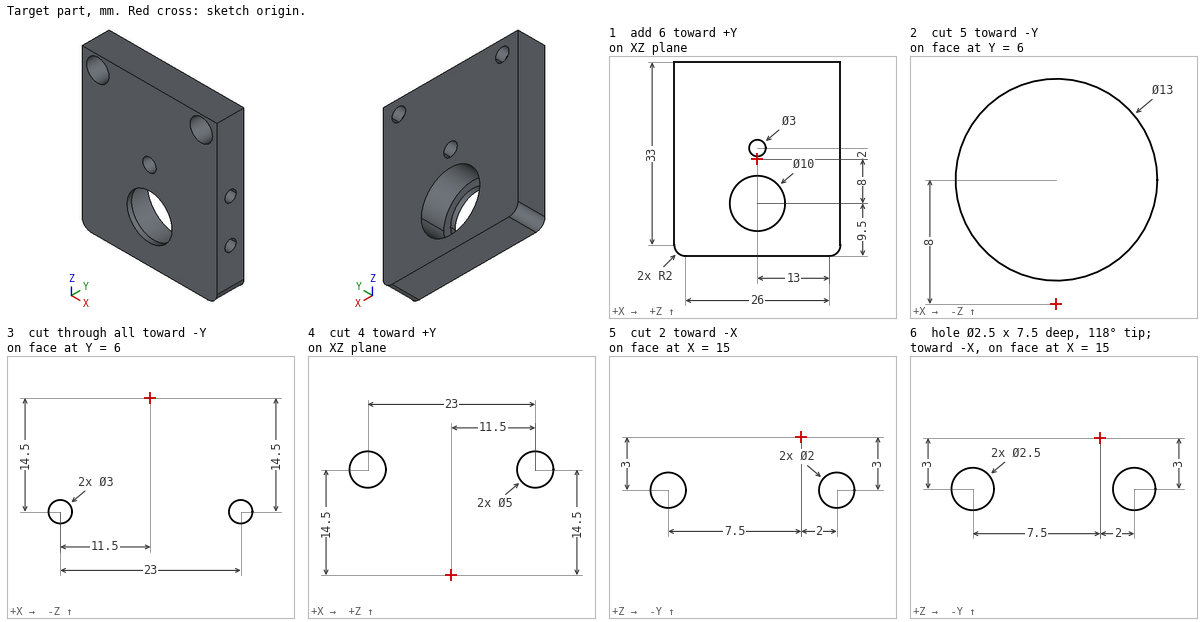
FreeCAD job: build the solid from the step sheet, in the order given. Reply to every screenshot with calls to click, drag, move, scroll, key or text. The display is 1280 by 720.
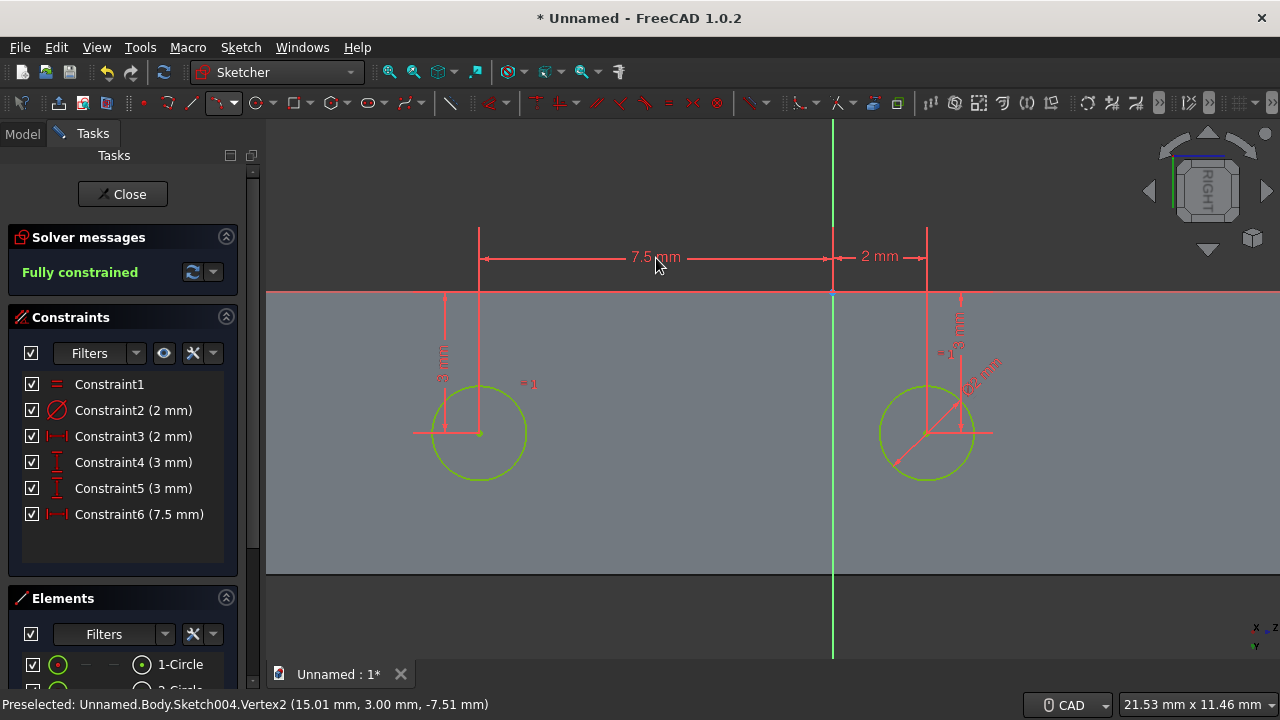
click(123, 194)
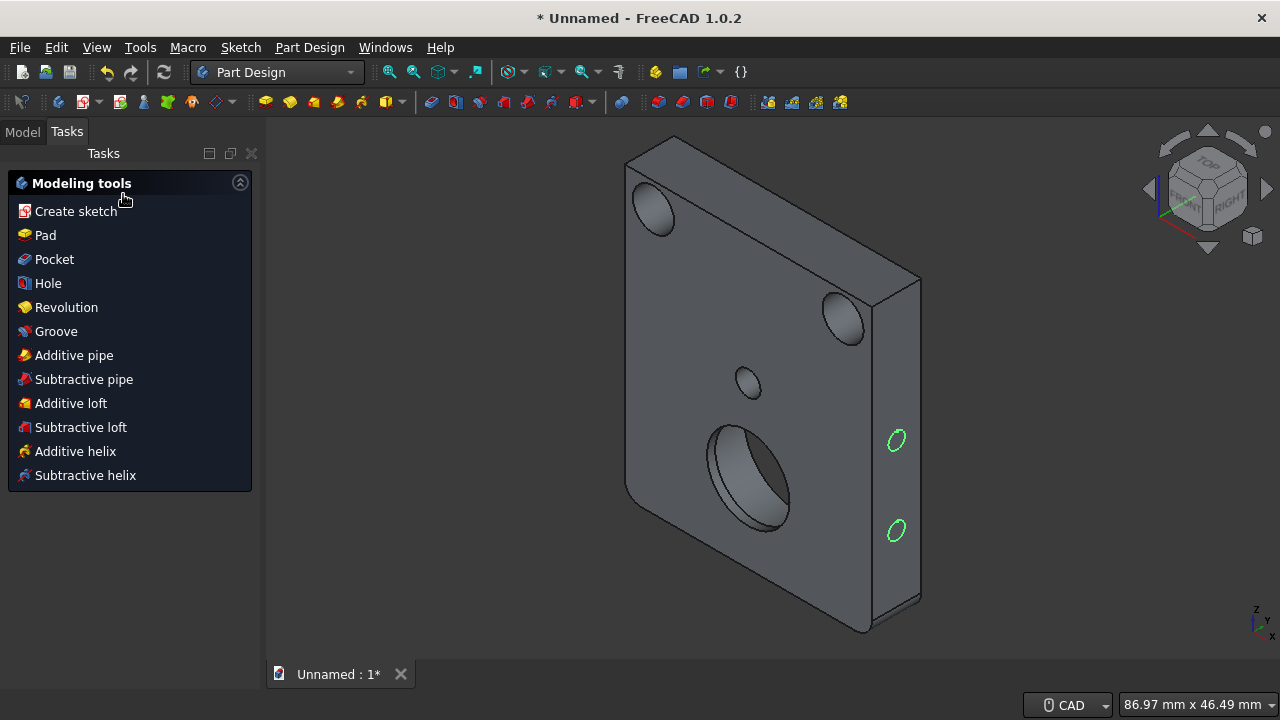
click(432, 102)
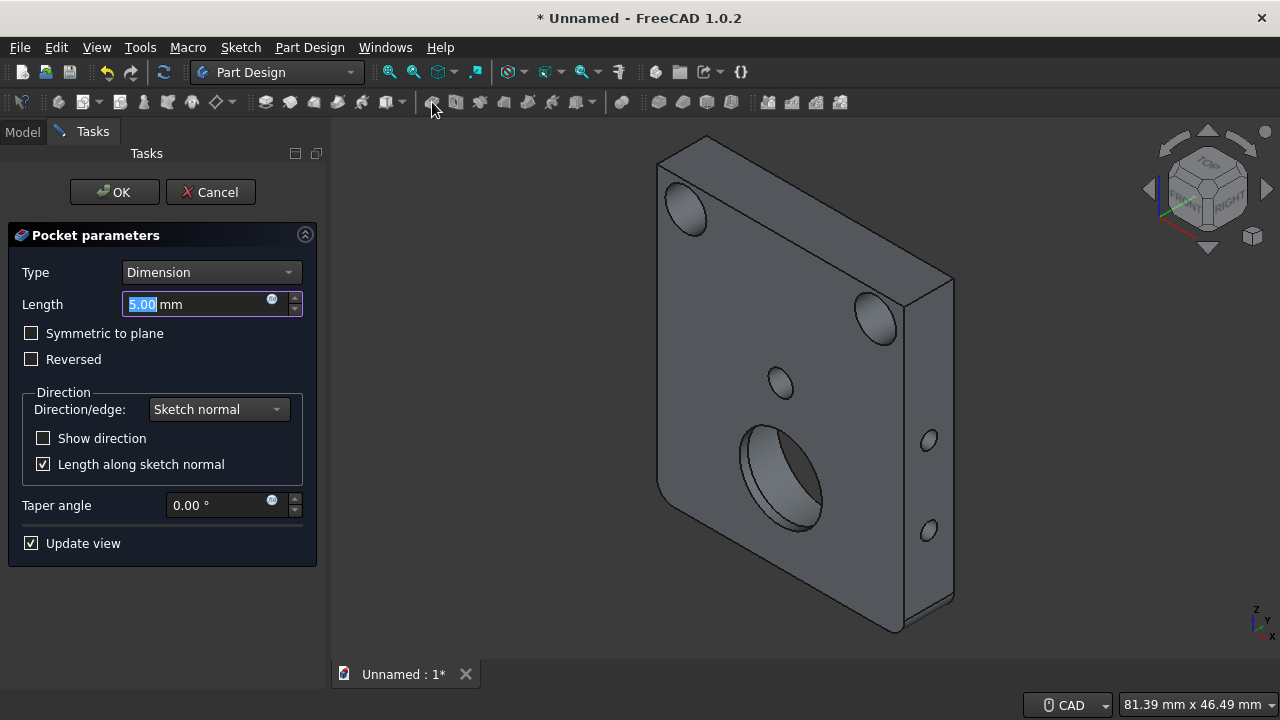
text(2)
key(Tab)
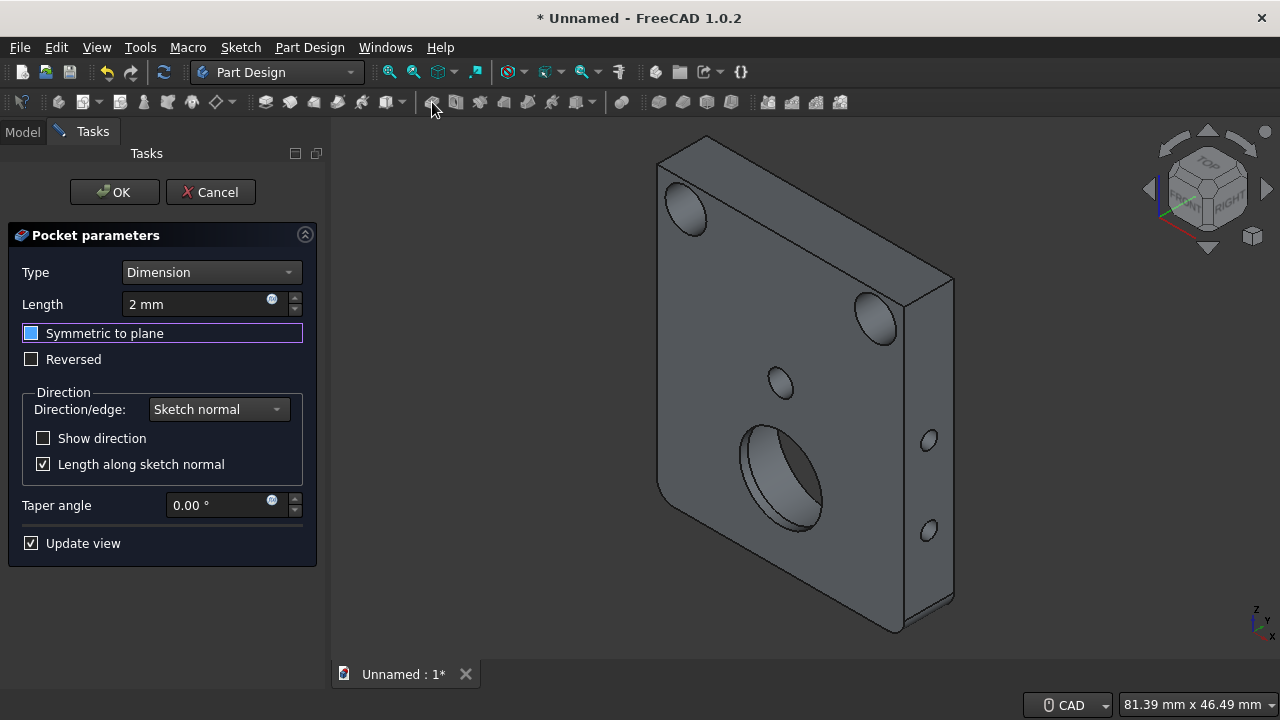
click(115, 192)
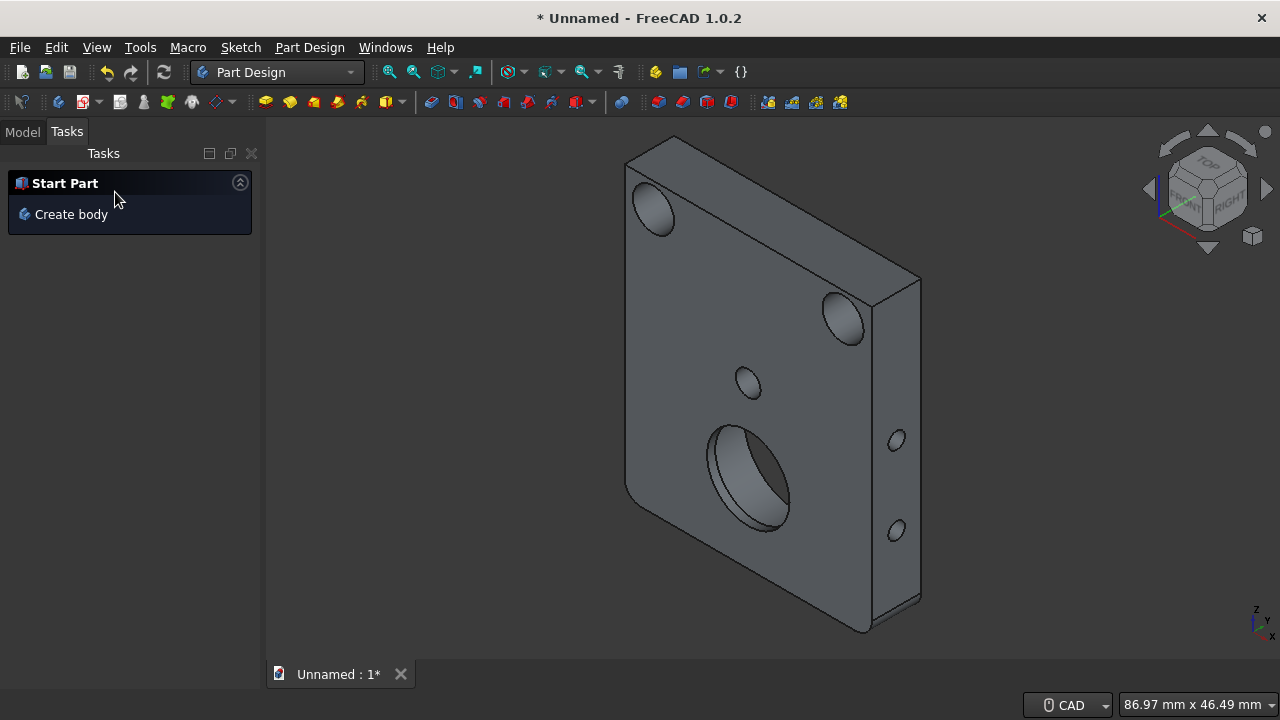
click(897, 359)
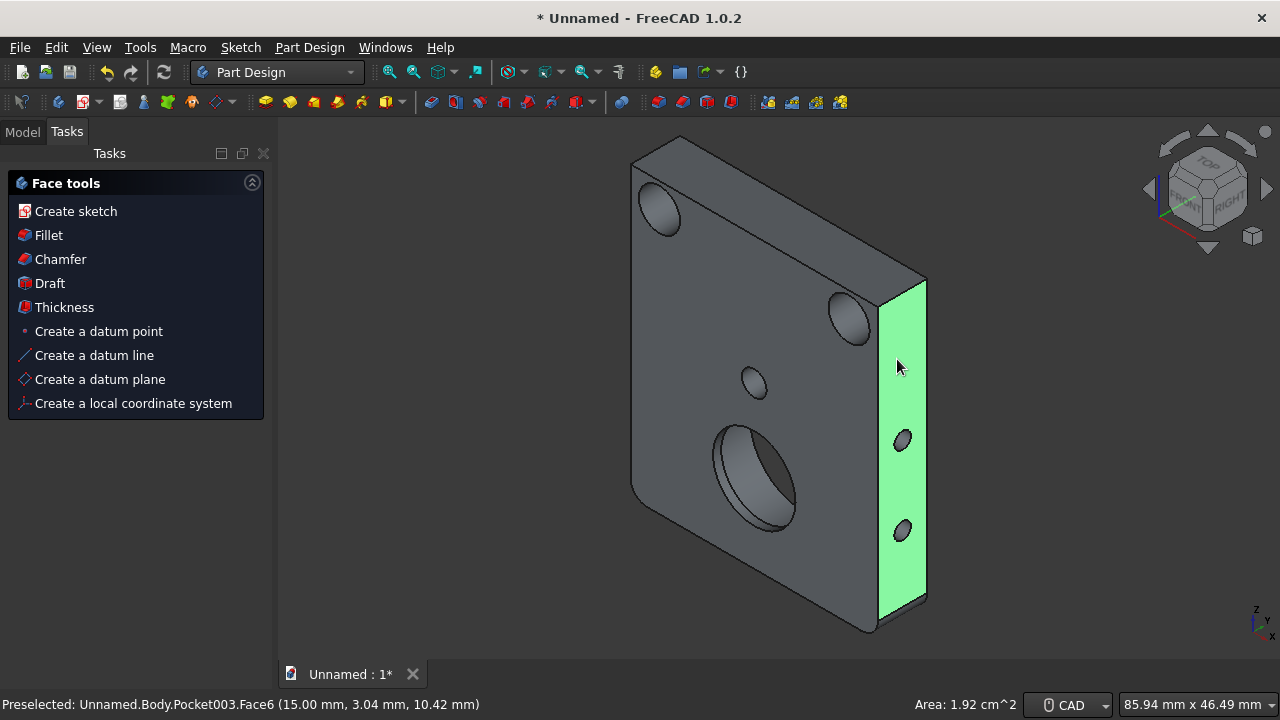
click(84, 102)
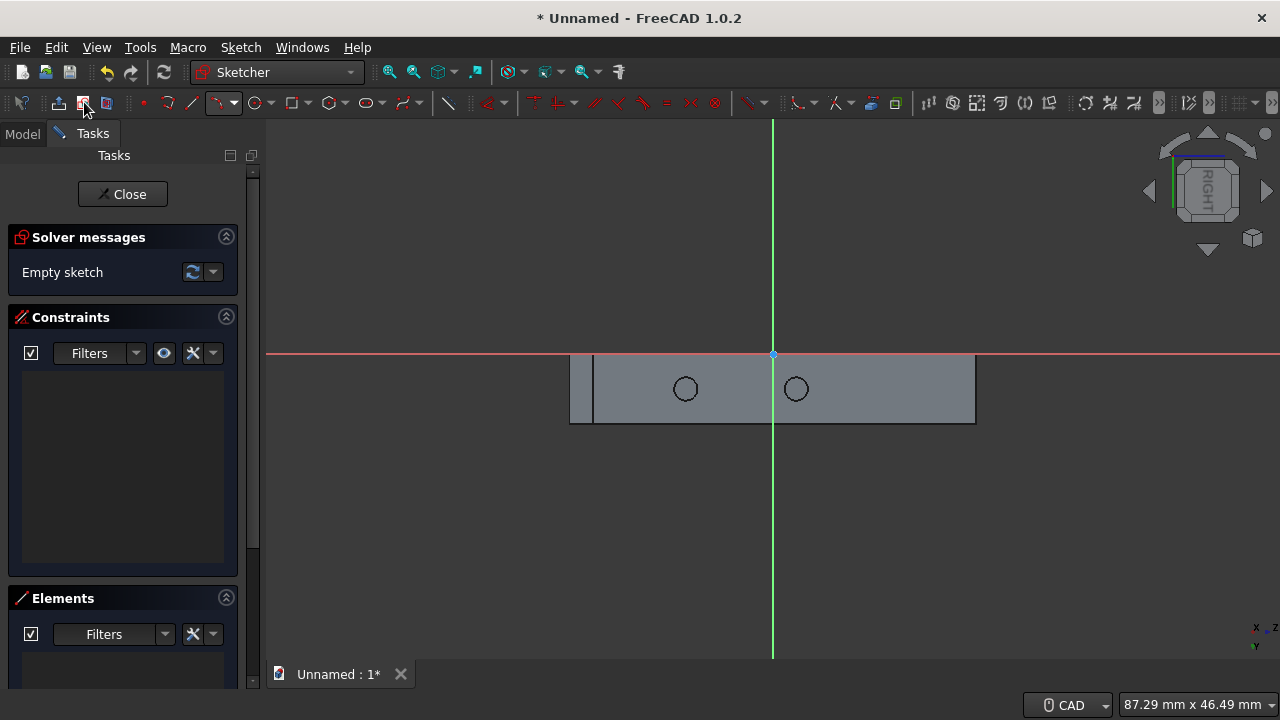
scroll(753, 376, up, 7)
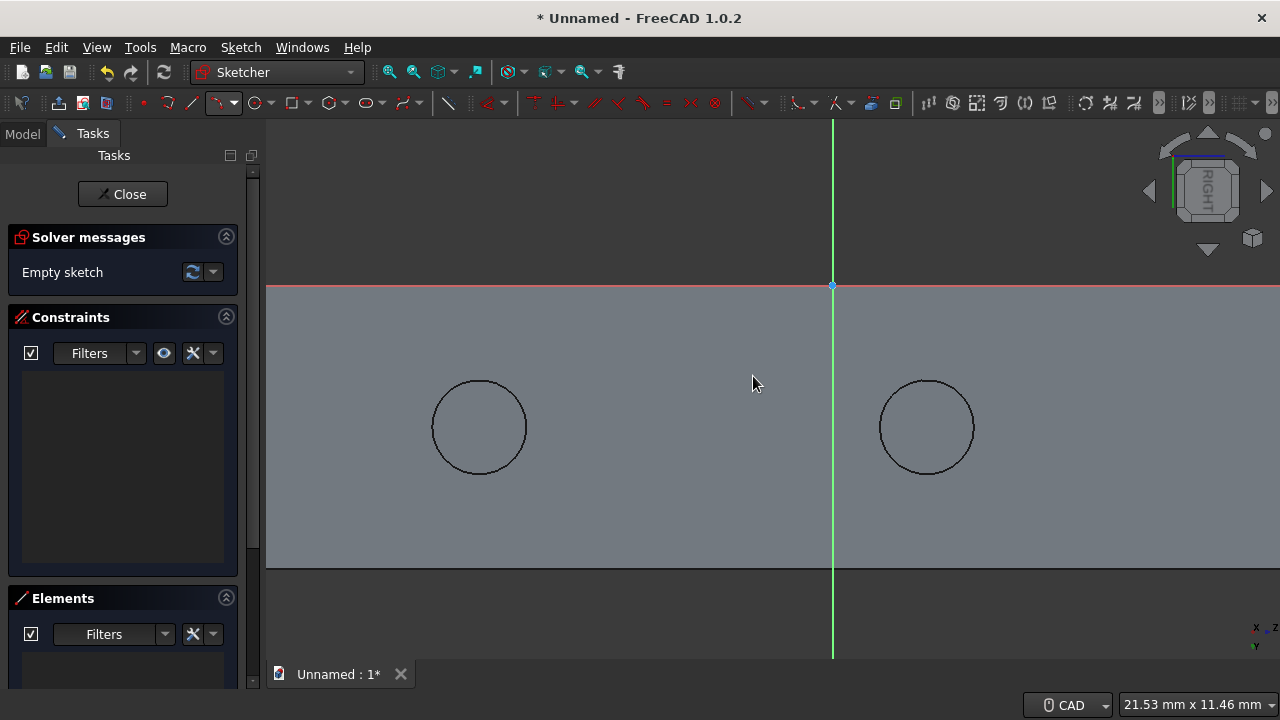
key(g)
key(c)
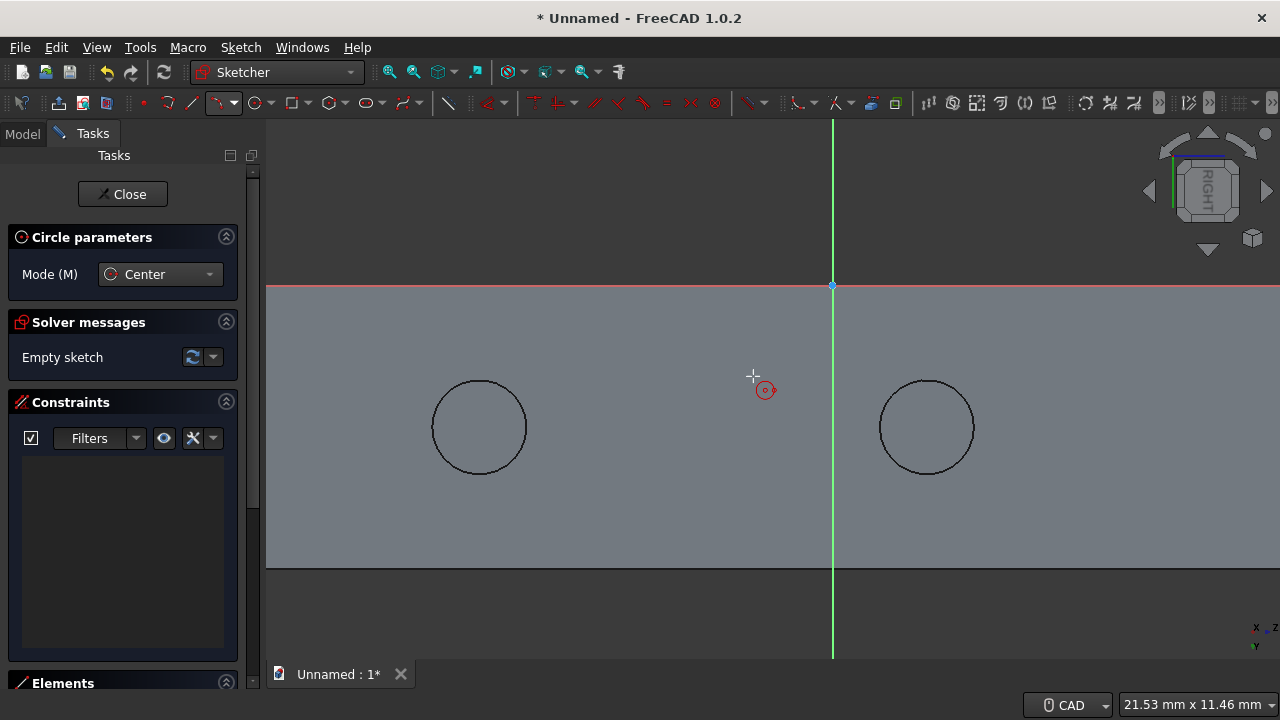
click(927, 427)
click(968, 386)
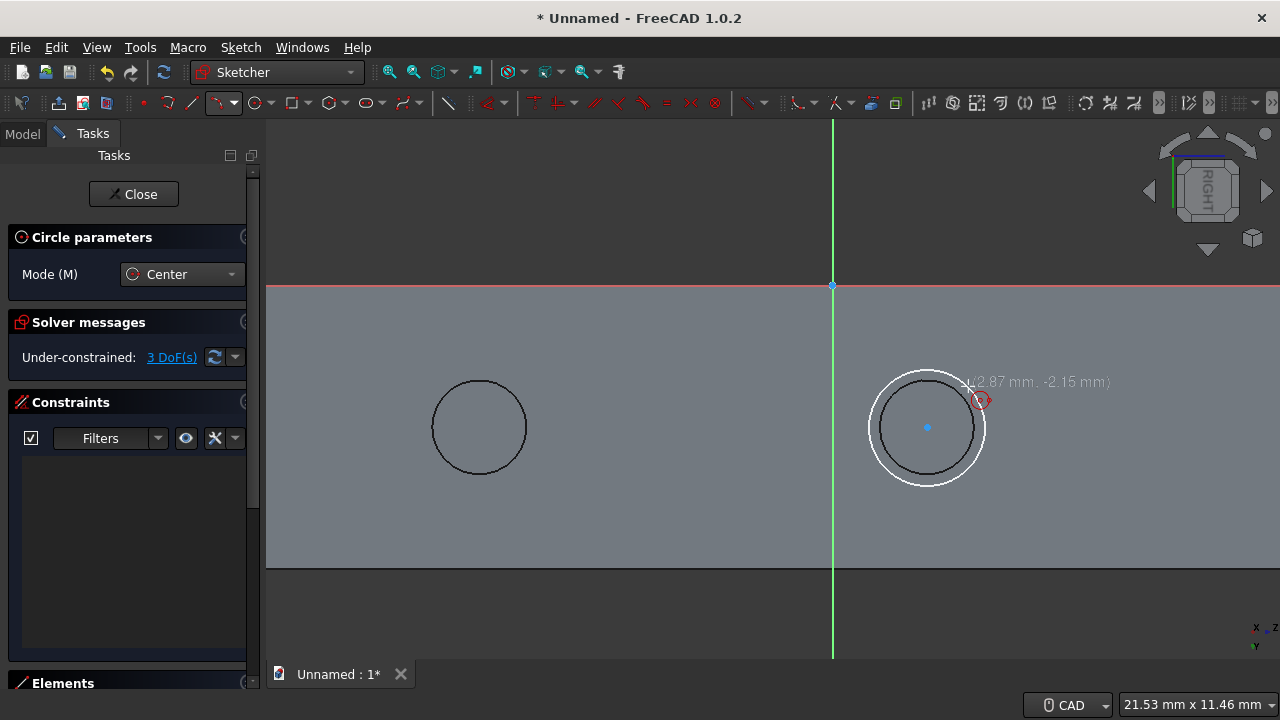
click(479, 427)
click(521, 386)
key(Escape)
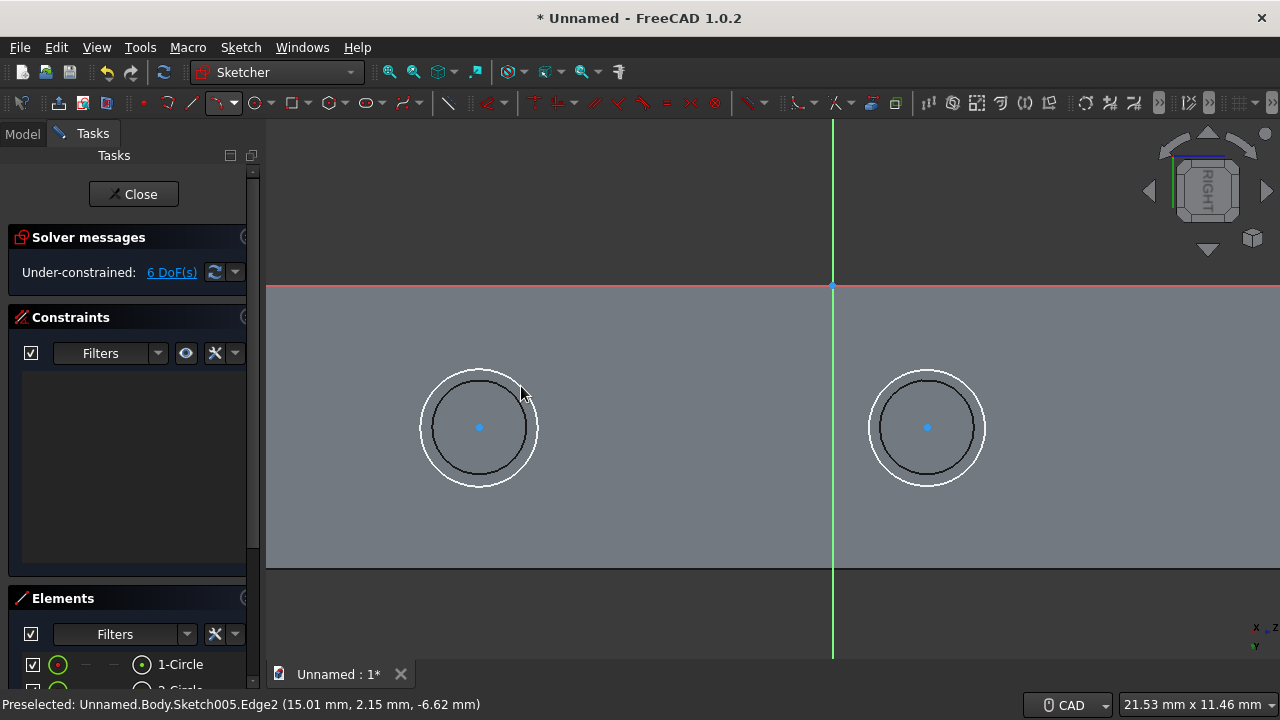
click(968, 387)